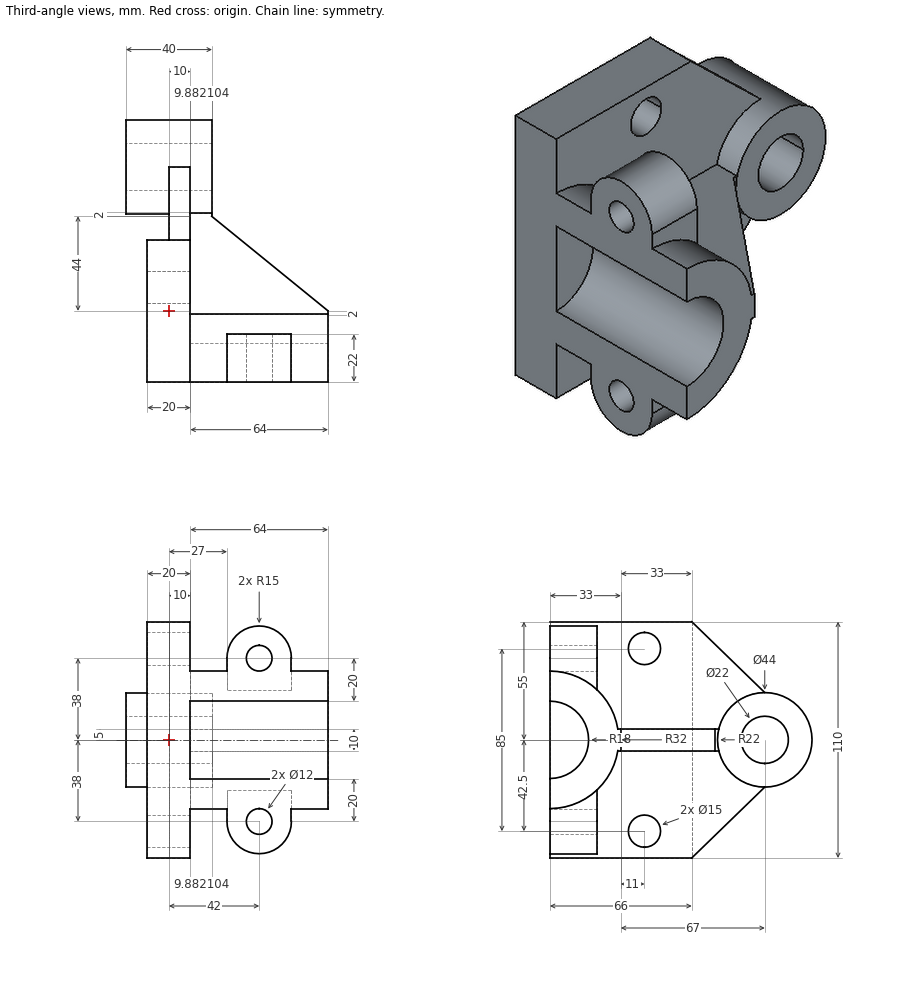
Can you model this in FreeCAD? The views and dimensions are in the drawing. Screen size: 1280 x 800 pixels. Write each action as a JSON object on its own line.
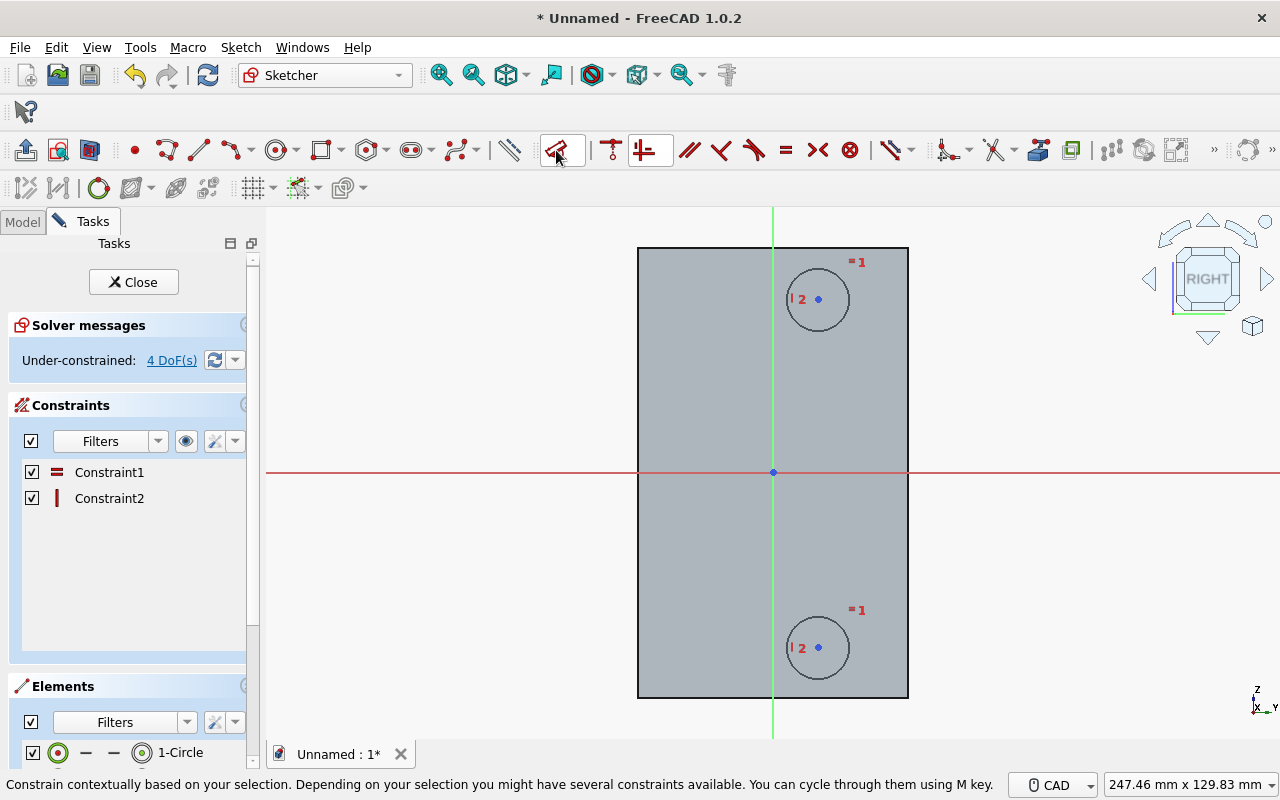
{"action": "left_click", "coordinate": [840, 626]}
{"action": "left_click", "coordinate": [863, 603]}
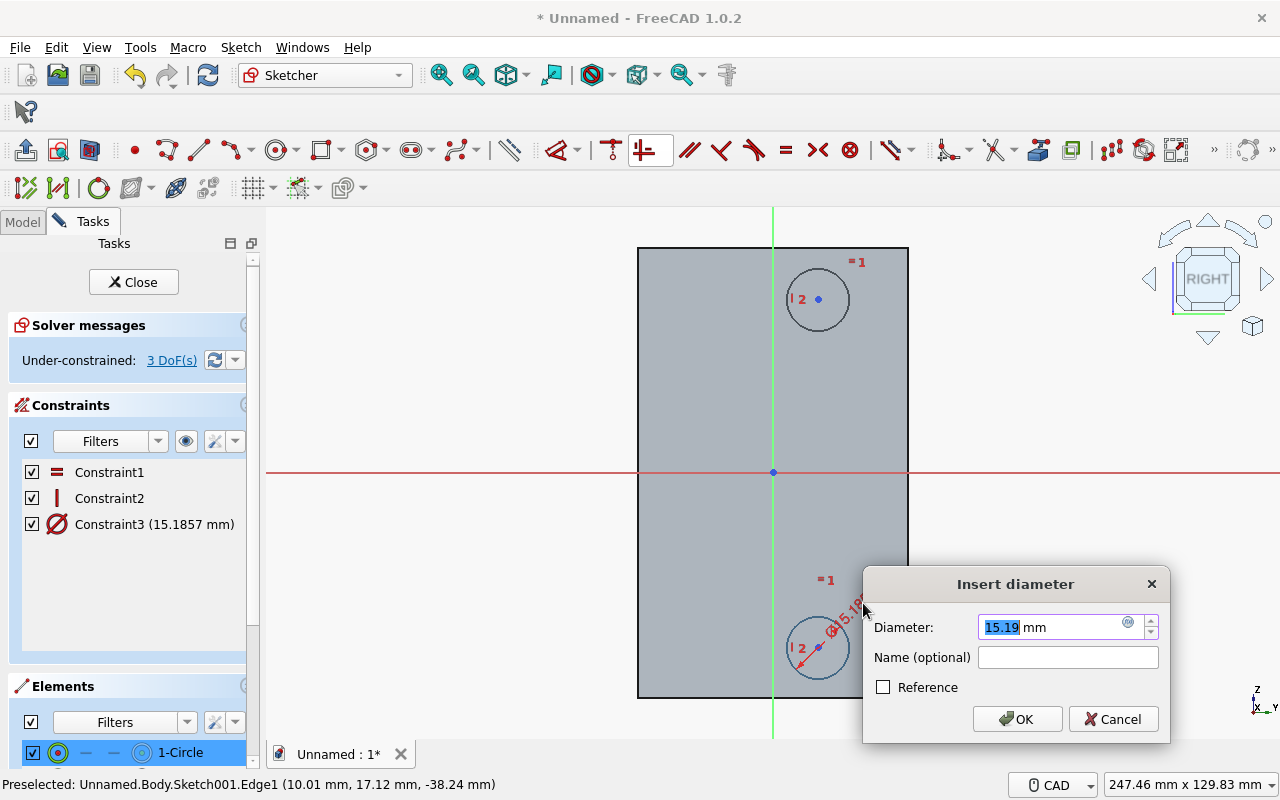
{"action": "type", "text": "15"}
{"action": "key", "text": "Return"}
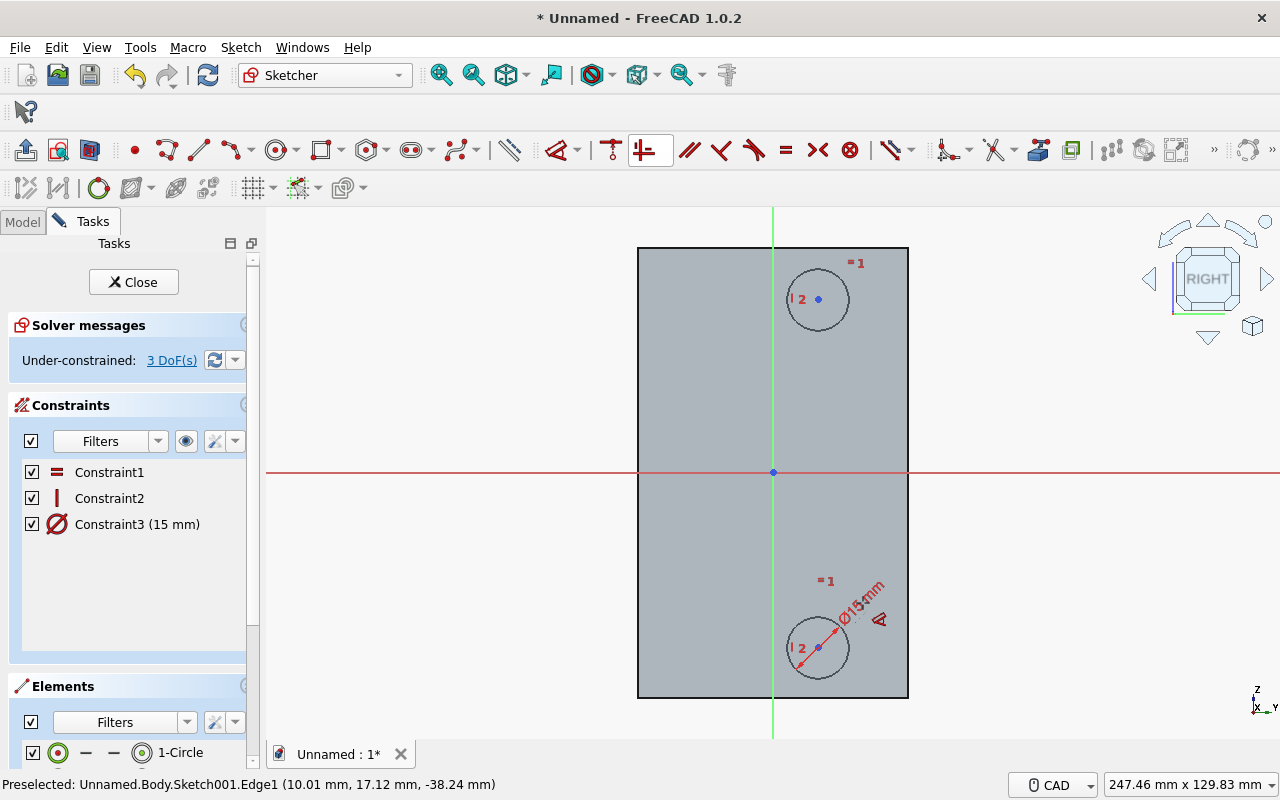
{"action": "left_click", "coordinate": [818, 648]}
{"action": "left_click", "coordinate": [795, 439]}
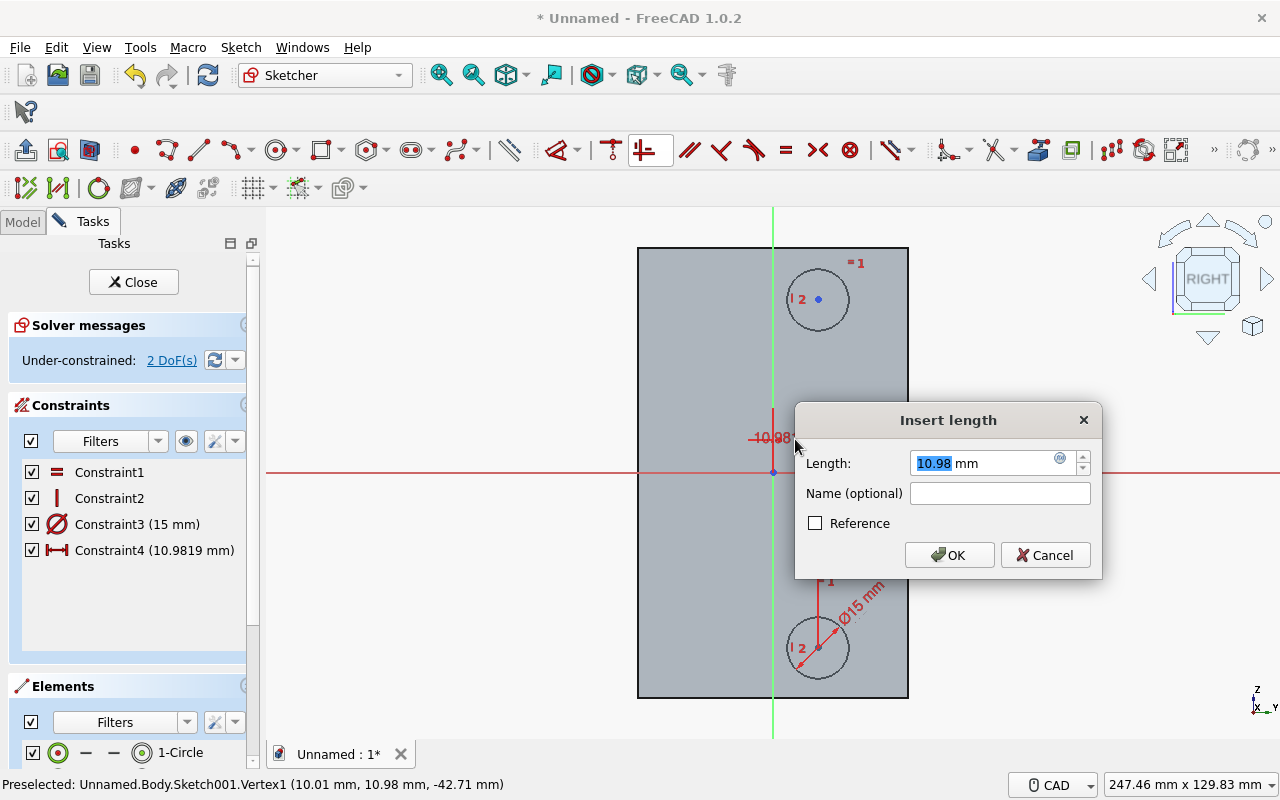
{"action": "type", "text": "11"}
{"action": "key", "text": "Return"}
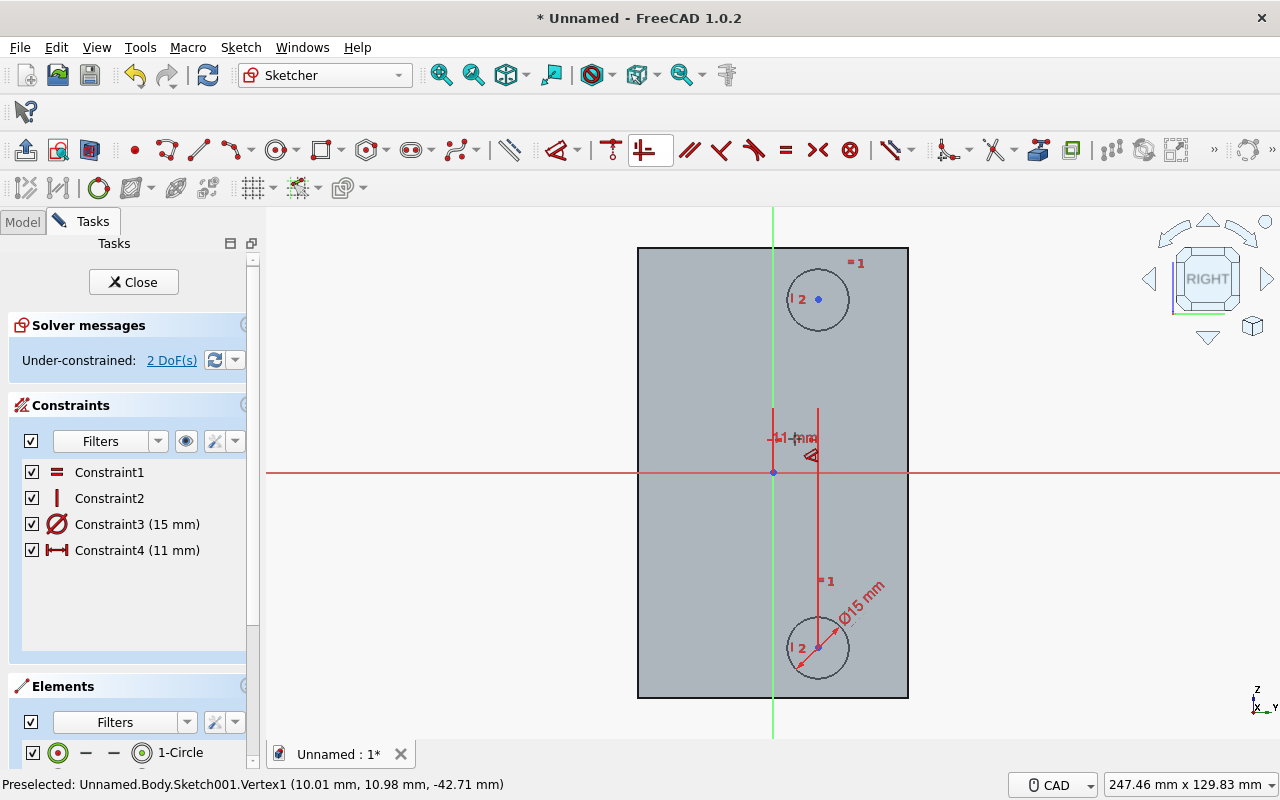
{"action": "left_click", "coordinate": [818, 648]}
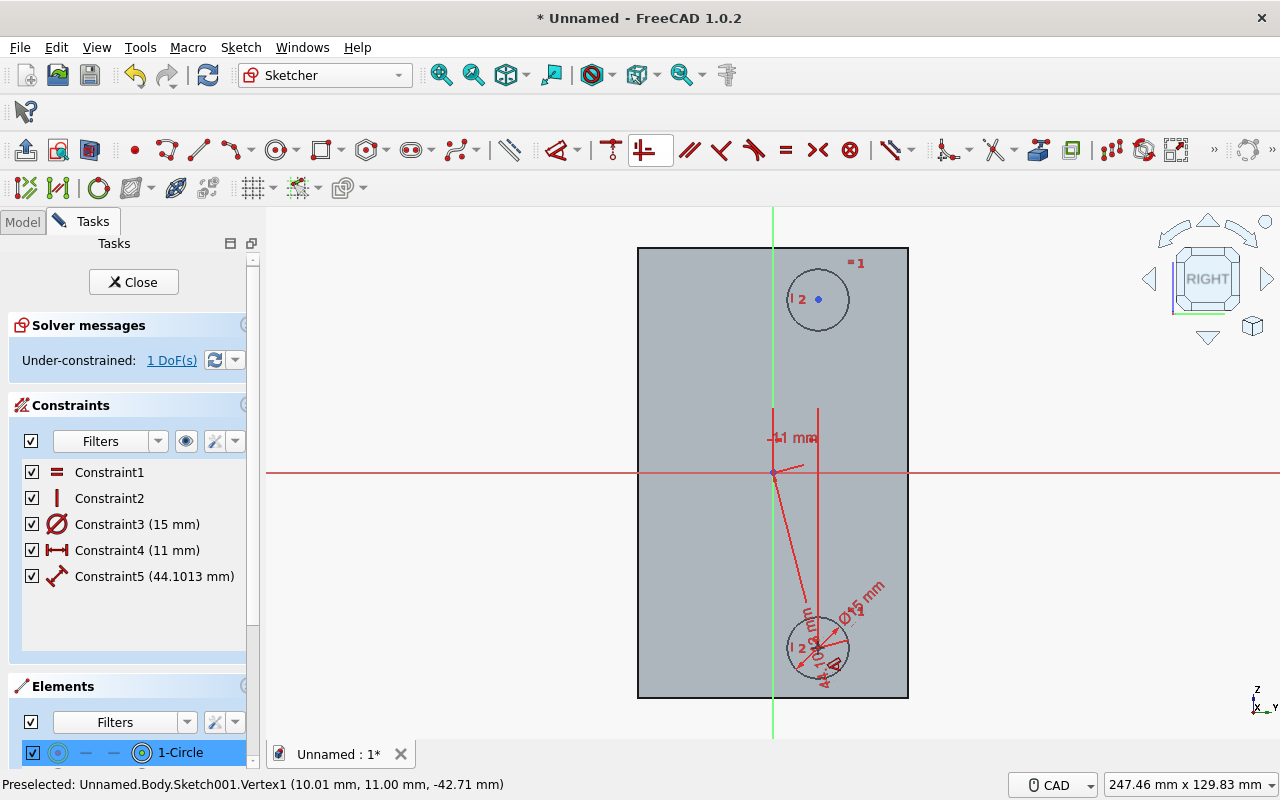
{"action": "left_click", "coordinate": [818, 300]}
{"action": "left_click", "coordinate": [852, 394]}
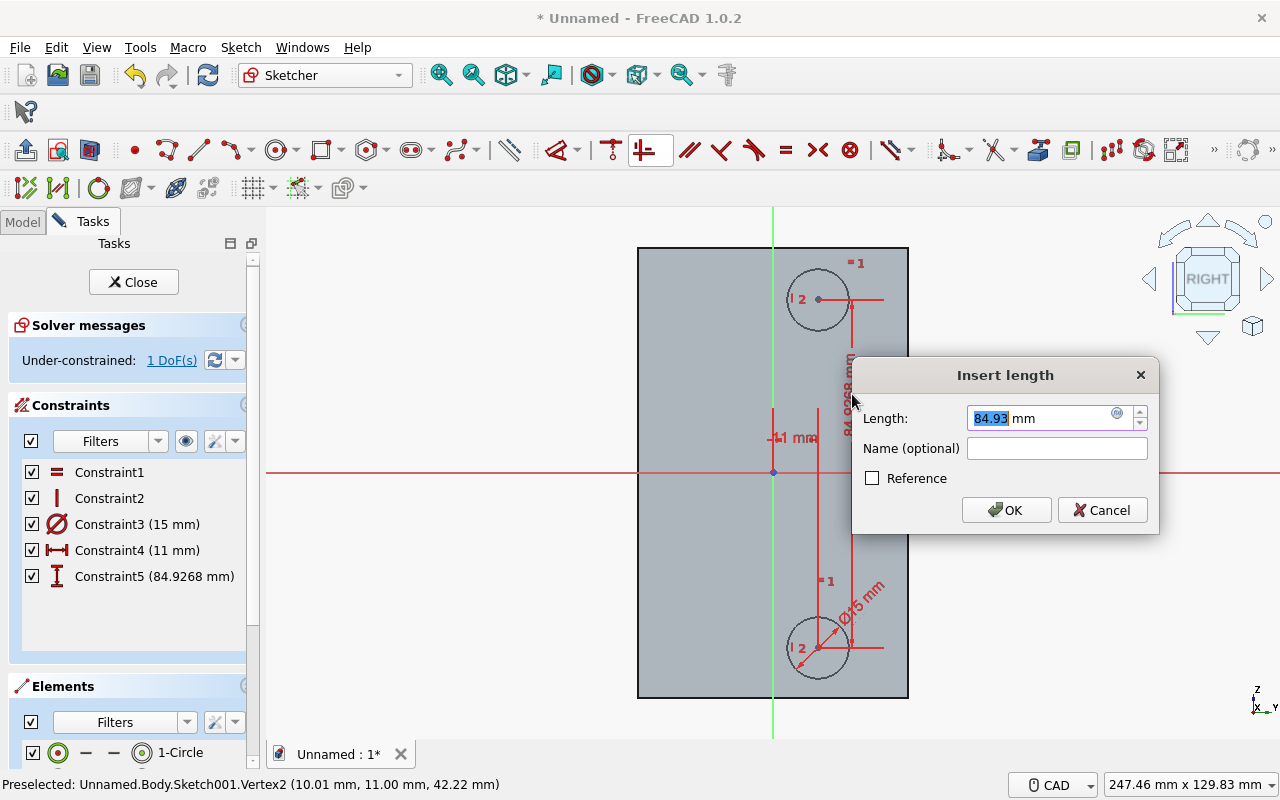
{"action": "type", "text": "85"}
{"action": "key", "text": "Return"}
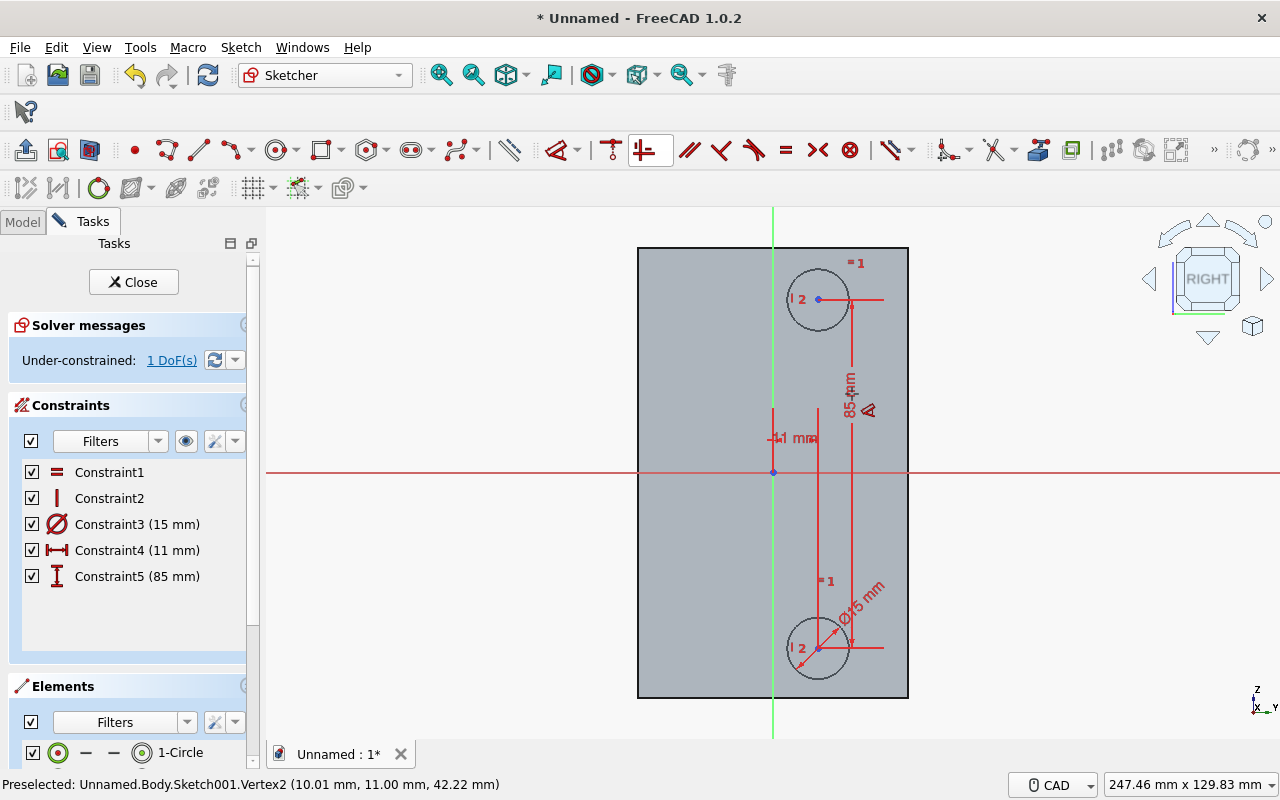
{"action": "left_click", "coordinate": [818, 648]}
{"action": "left_click", "coordinate": [739, 561]}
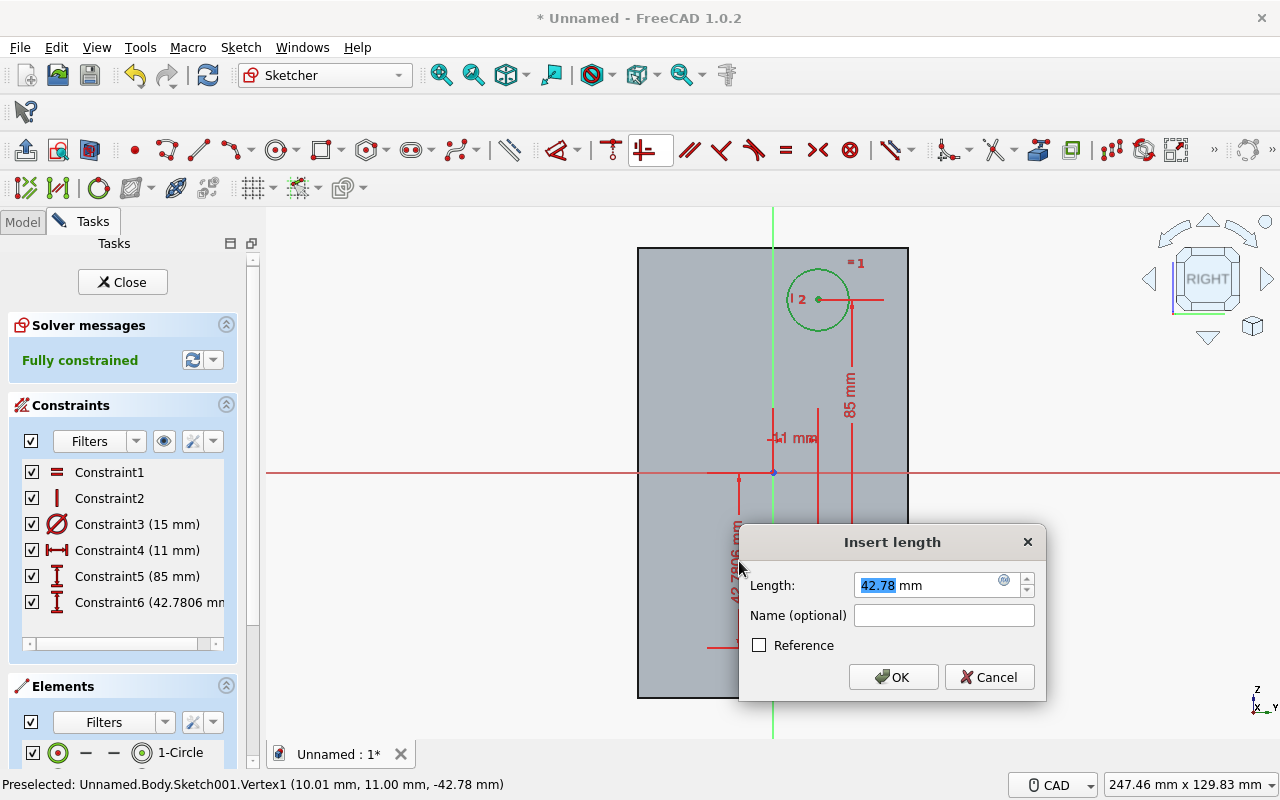
{"action": "type", "text": "42.5"}
{"action": "key", "text": "Return"}
{"action": "key", "text": "Escape"}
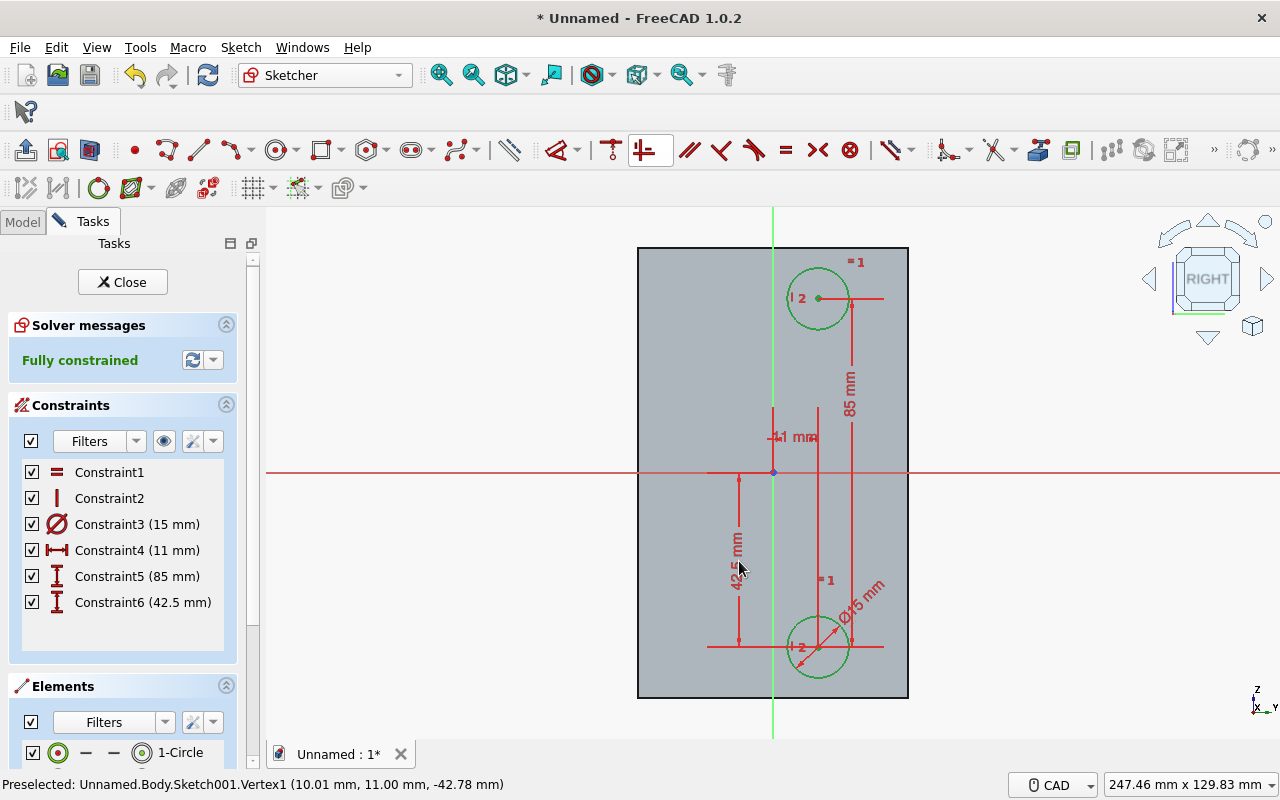
{"action": "left_click", "coordinate": [123, 282]}